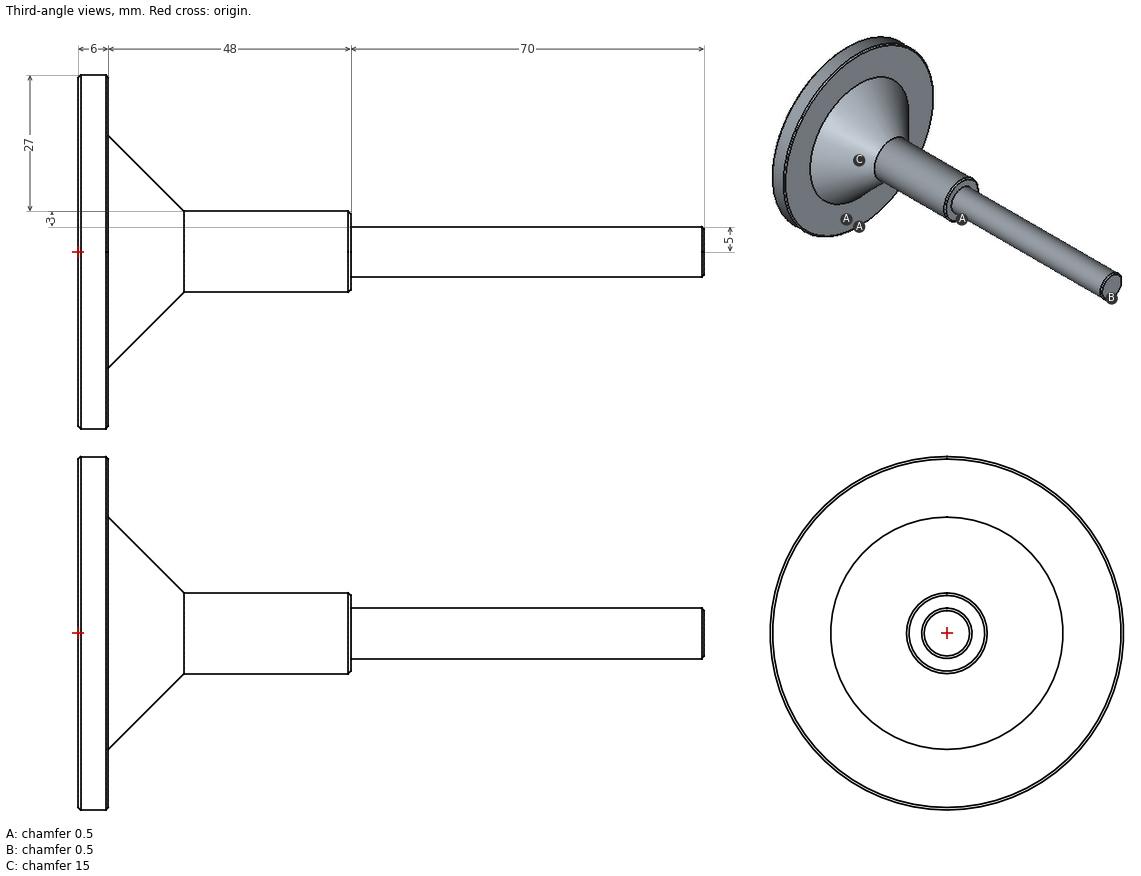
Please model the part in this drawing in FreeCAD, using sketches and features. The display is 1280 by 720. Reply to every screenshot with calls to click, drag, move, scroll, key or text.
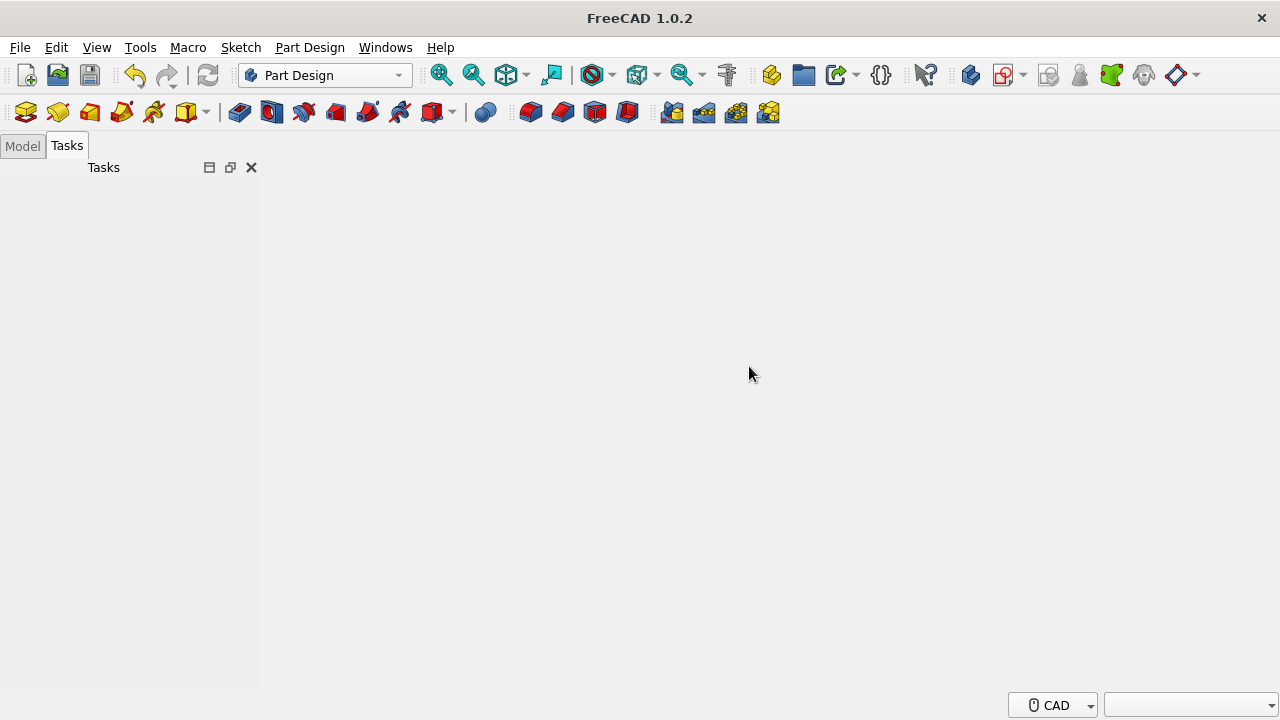
click(26, 76)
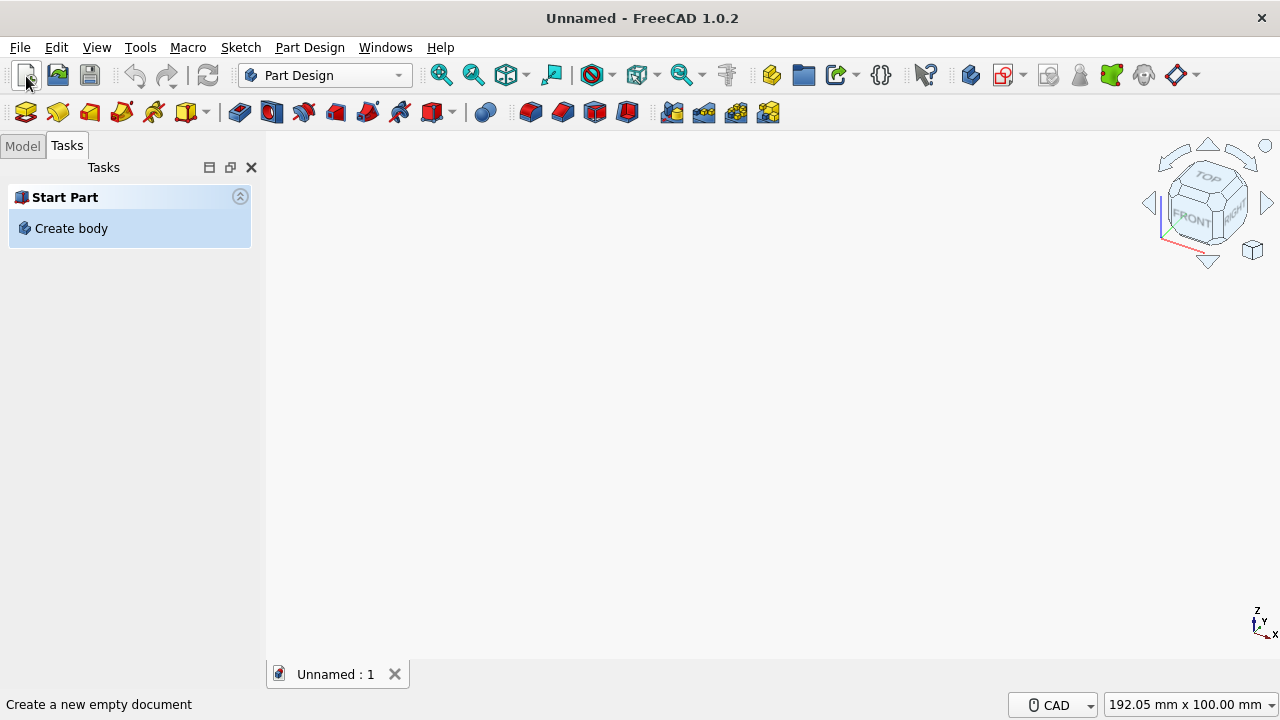
click(1004, 76)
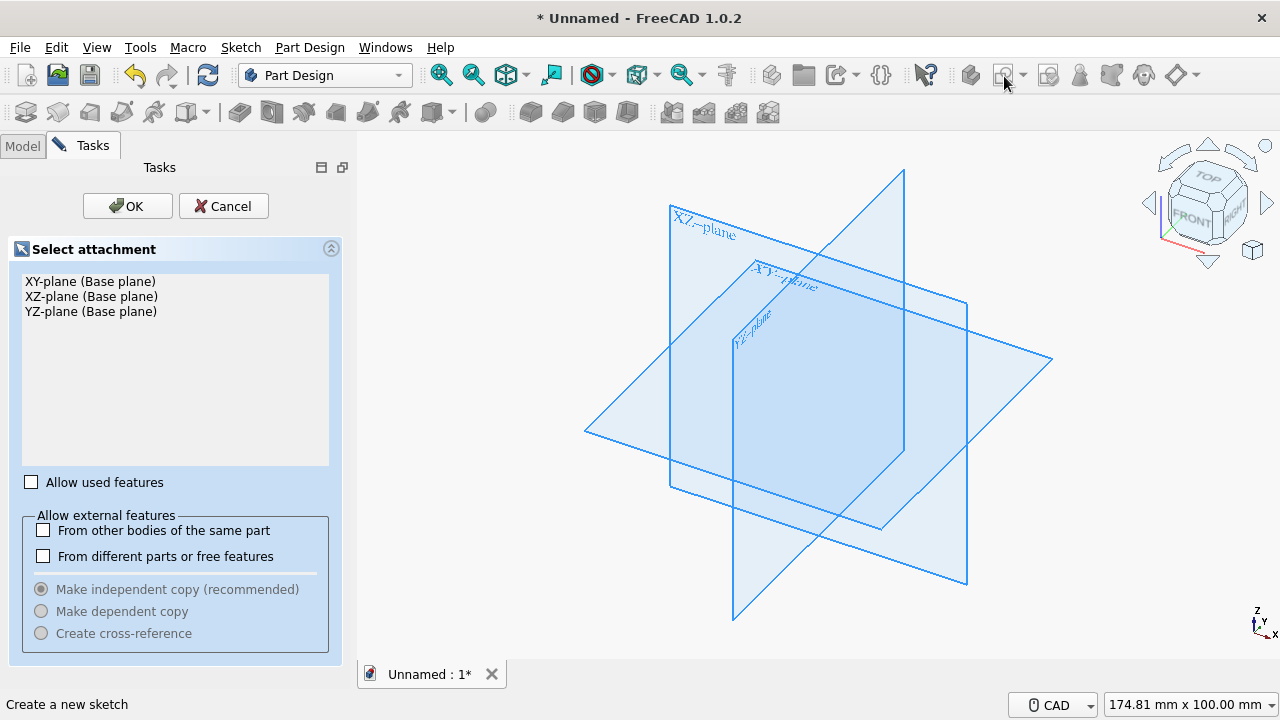
click(82, 282)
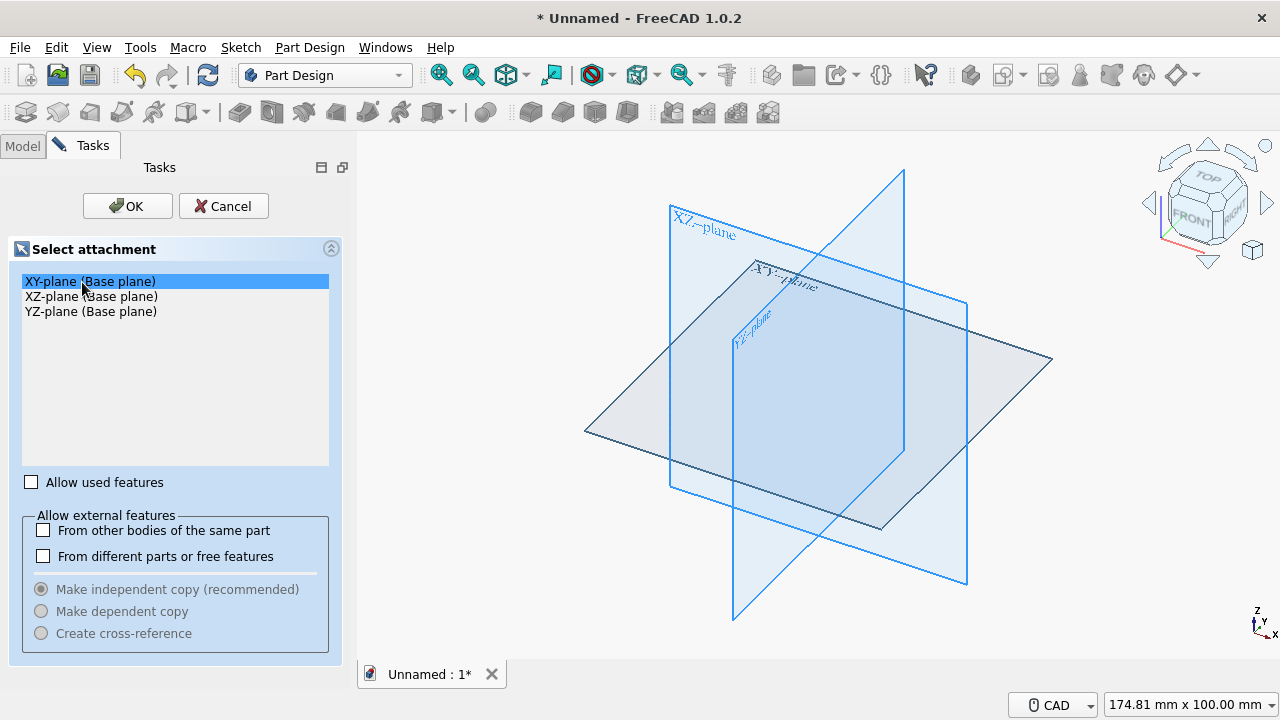
click(128, 206)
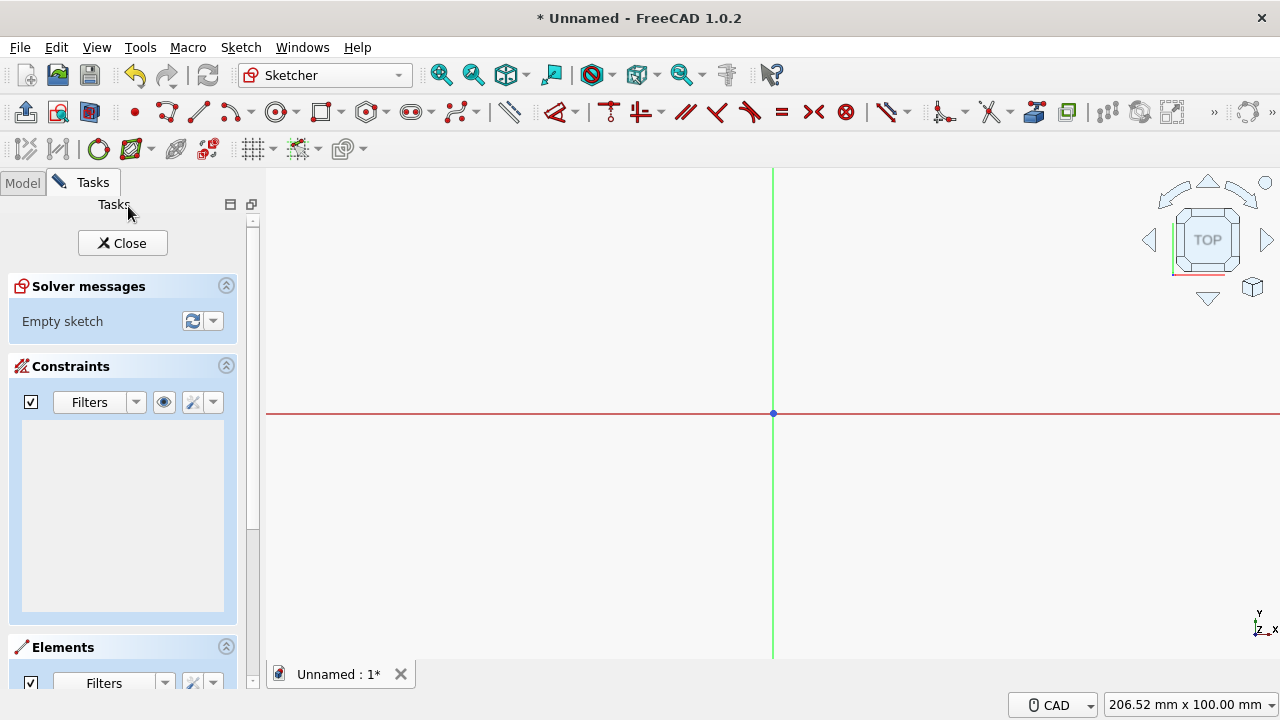
scroll(294, 588, down, 2)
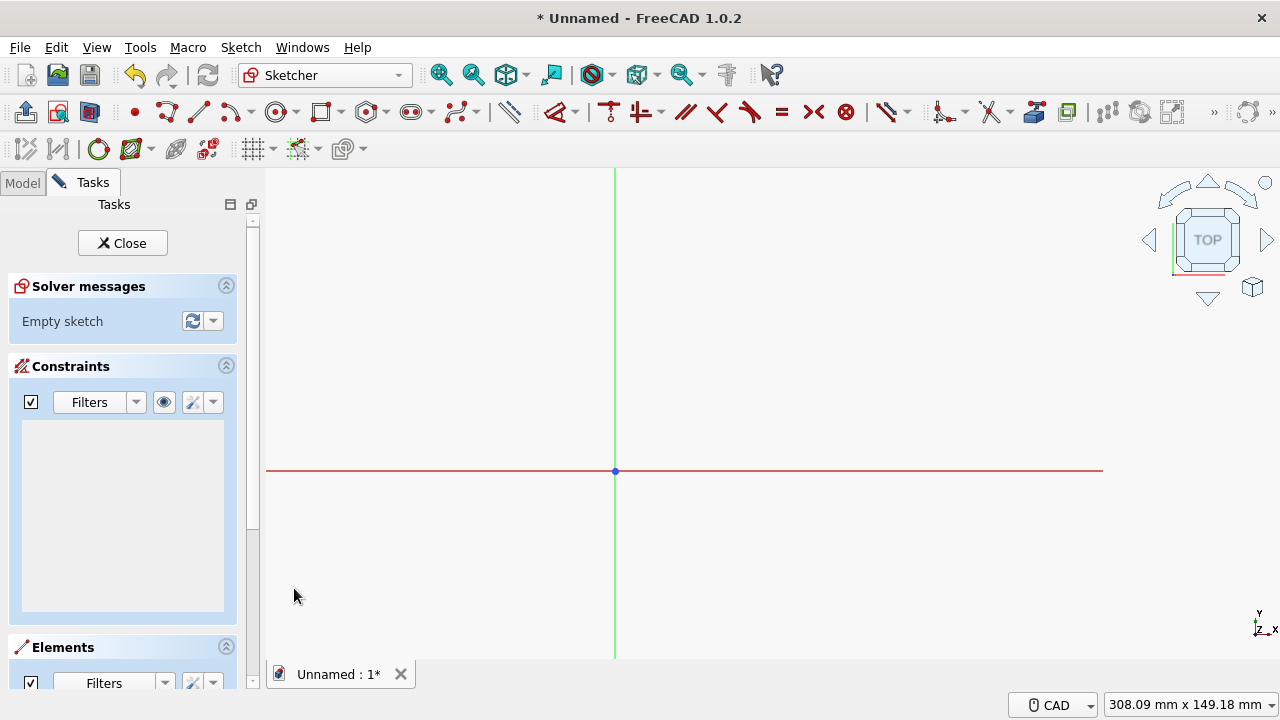
scroll(1052, 414, up, 2)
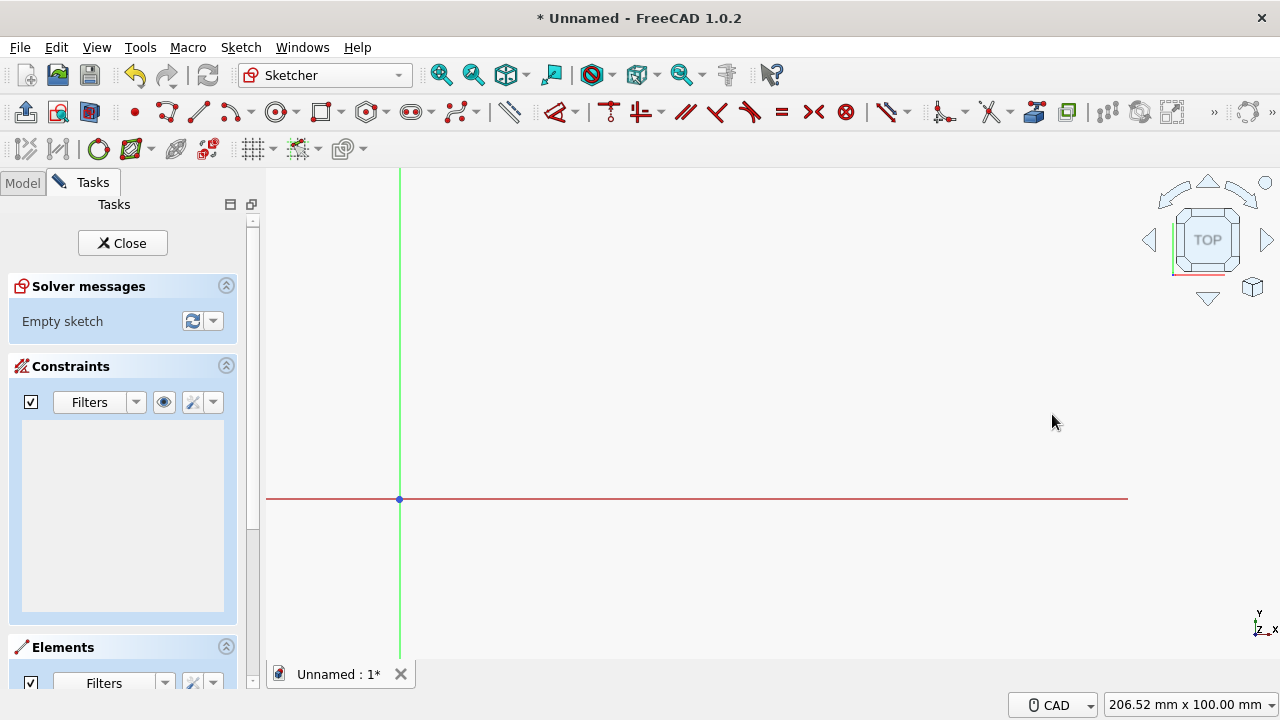
click(168, 112)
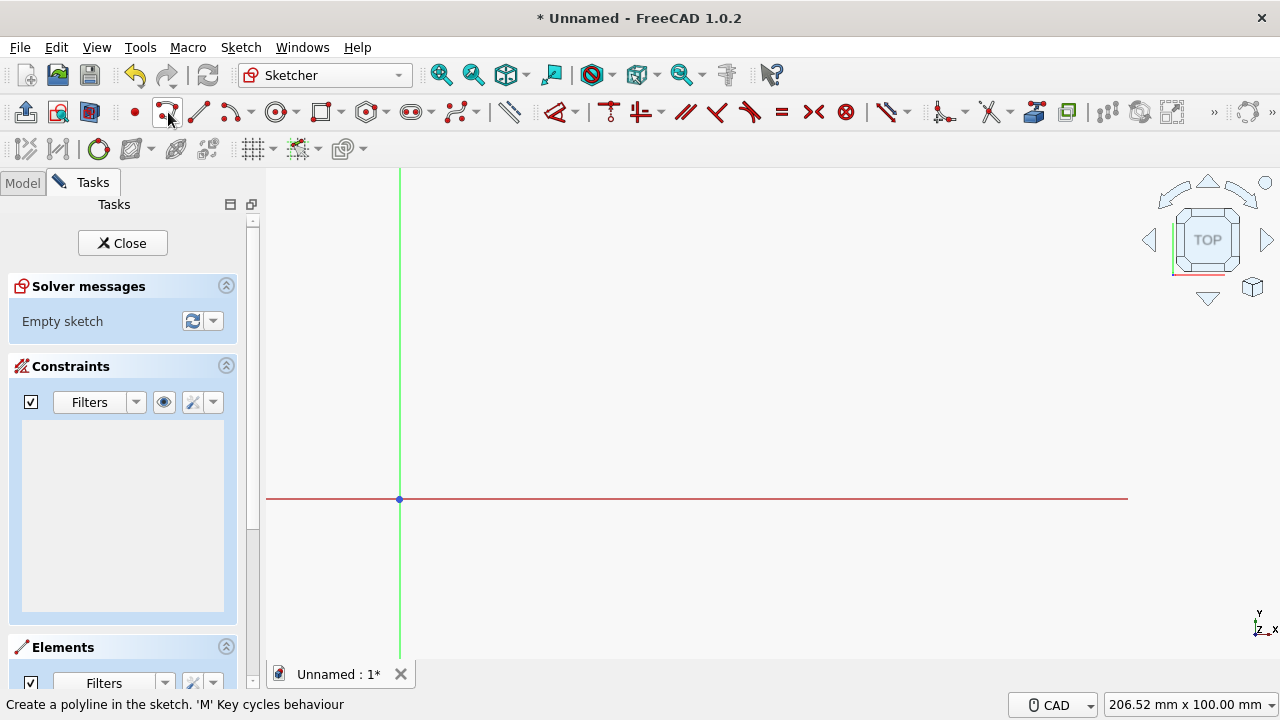
click(400, 499)
click(1009, 490)
click(1009, 475)
click(665, 475)
click(665, 460)
click(429, 460)
click(429, 327)
click(409, 327)
click(400, 499)
key(Escape)
key(Escape)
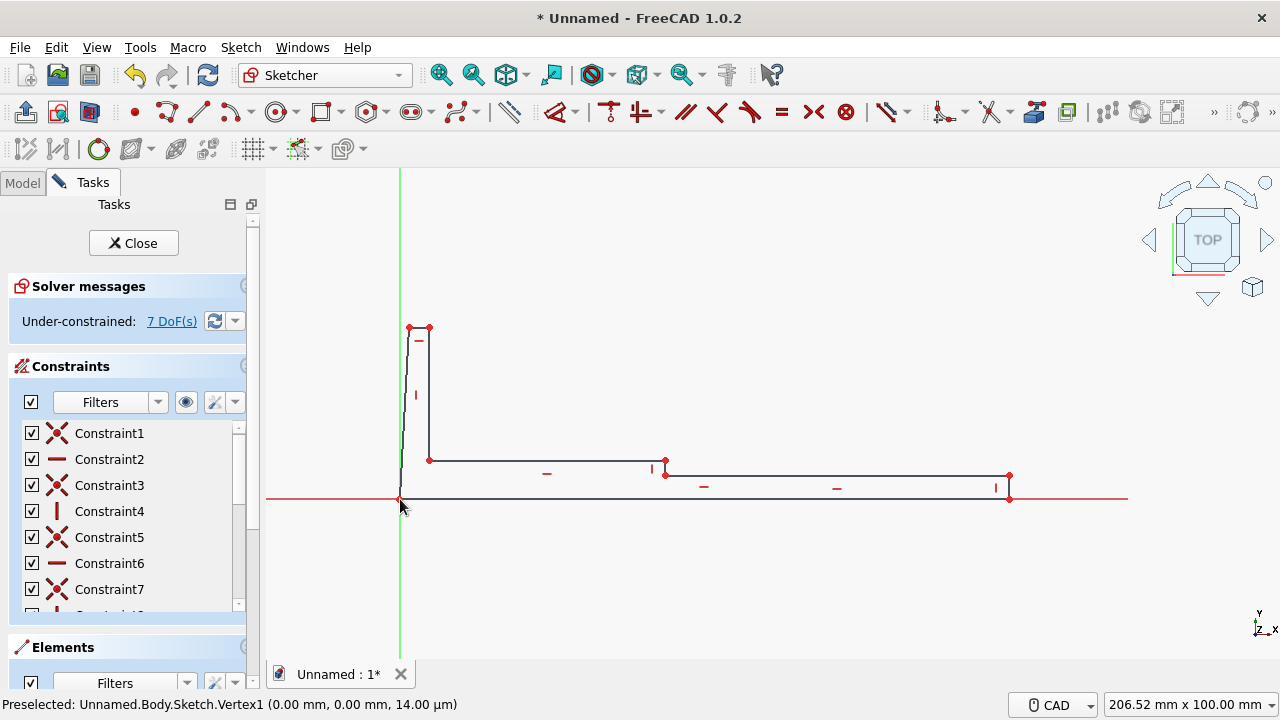
click(403, 448)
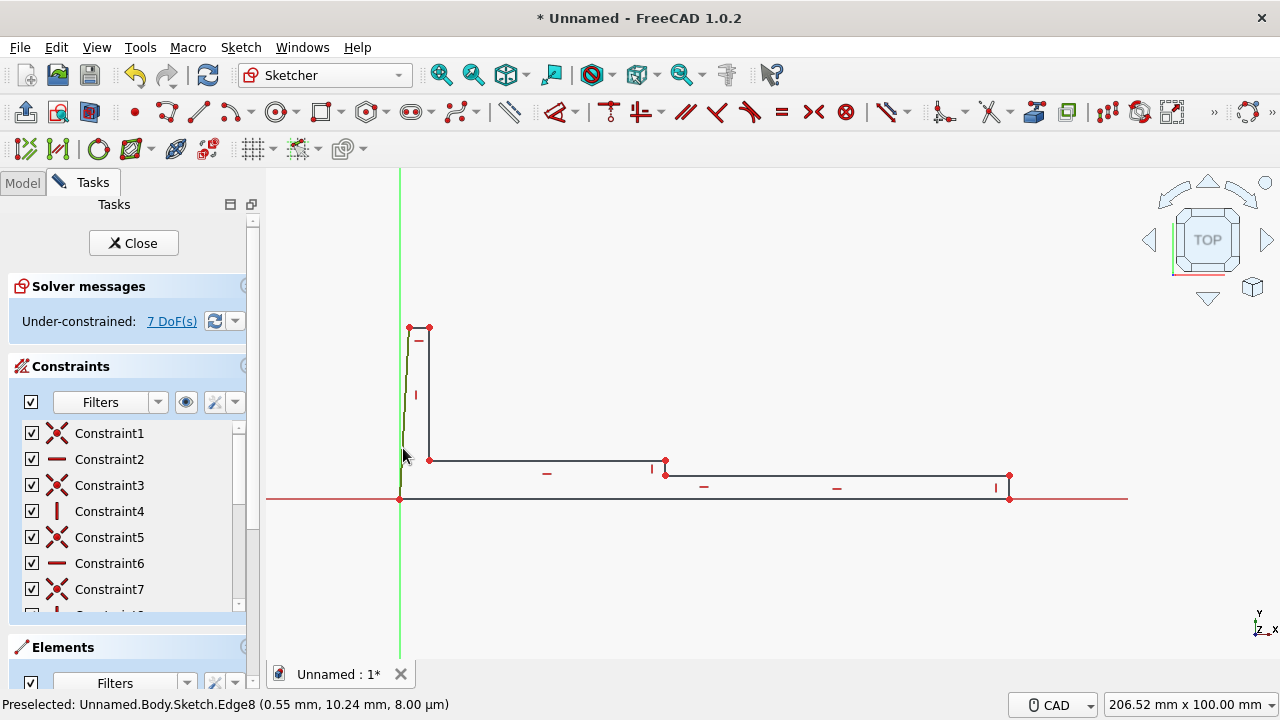
key(v)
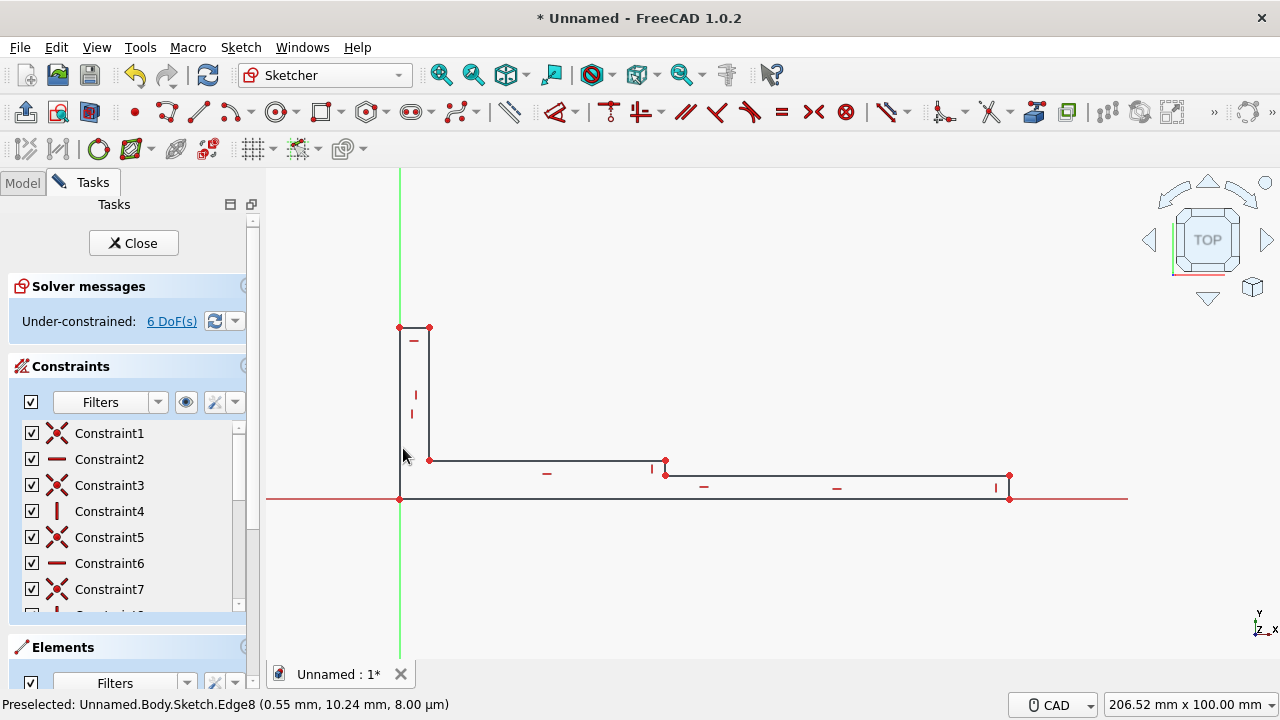
click(556, 112)